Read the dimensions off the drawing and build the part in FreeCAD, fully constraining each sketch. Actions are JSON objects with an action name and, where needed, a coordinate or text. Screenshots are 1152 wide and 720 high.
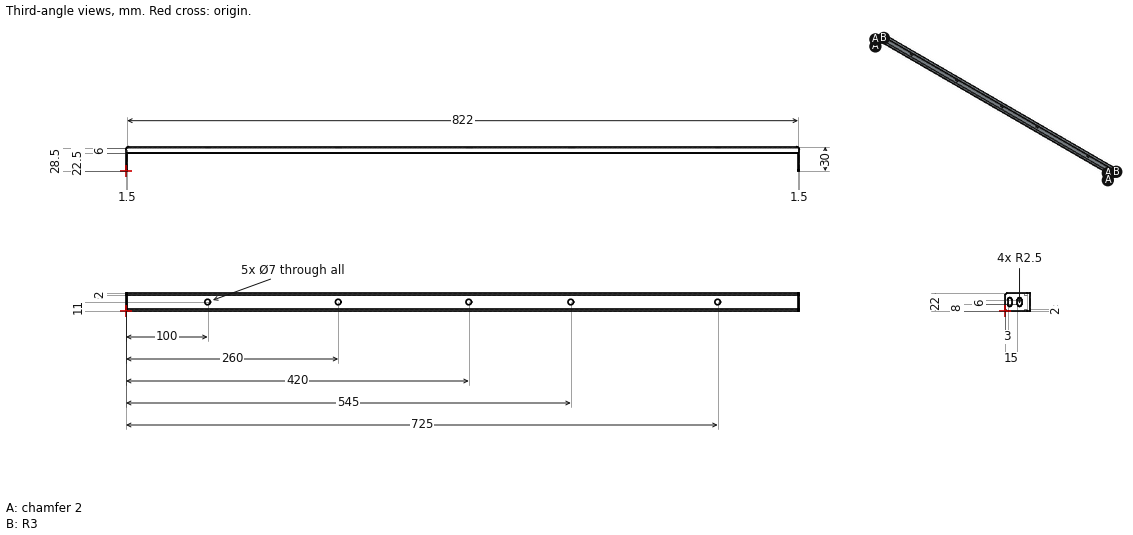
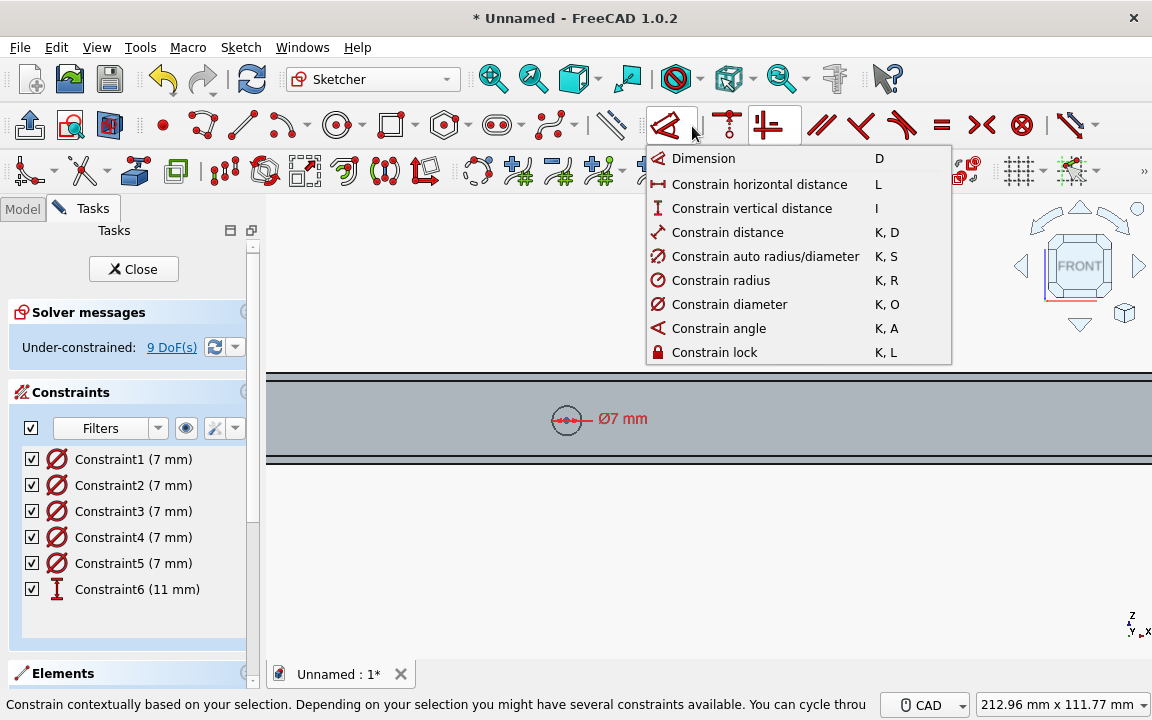
{"action": "left_click", "coordinate": [799, 208]}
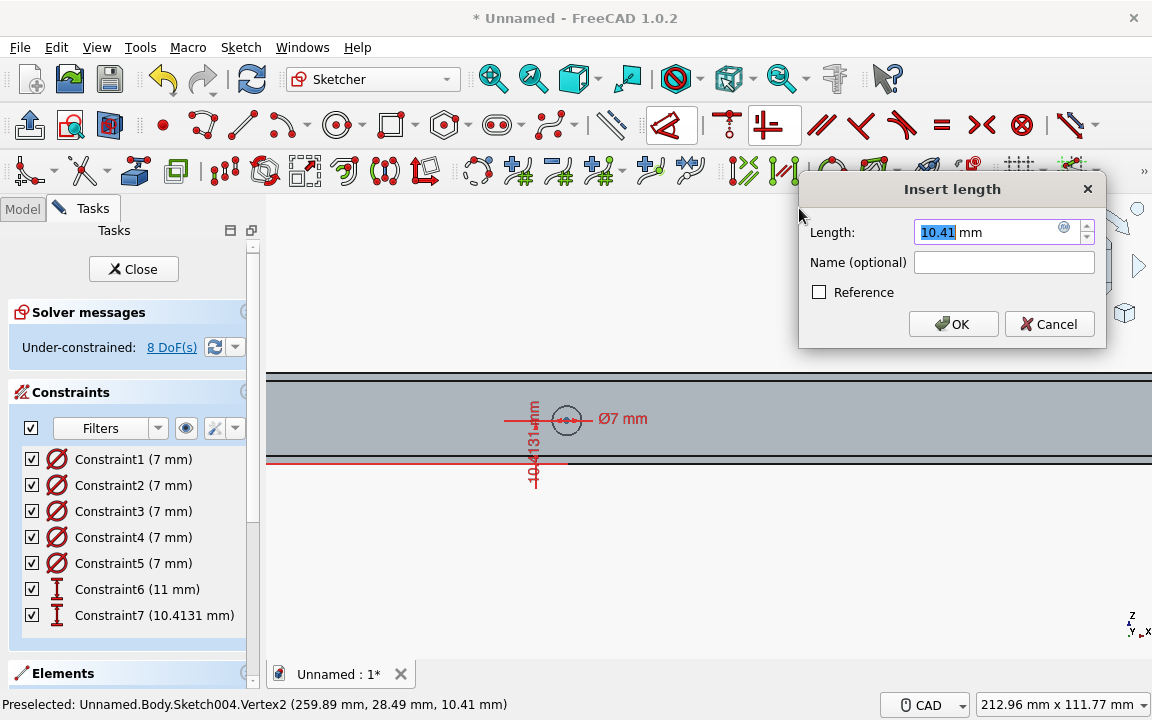
{"action": "type", "text": "11"}
{"action": "key", "text": "Return"}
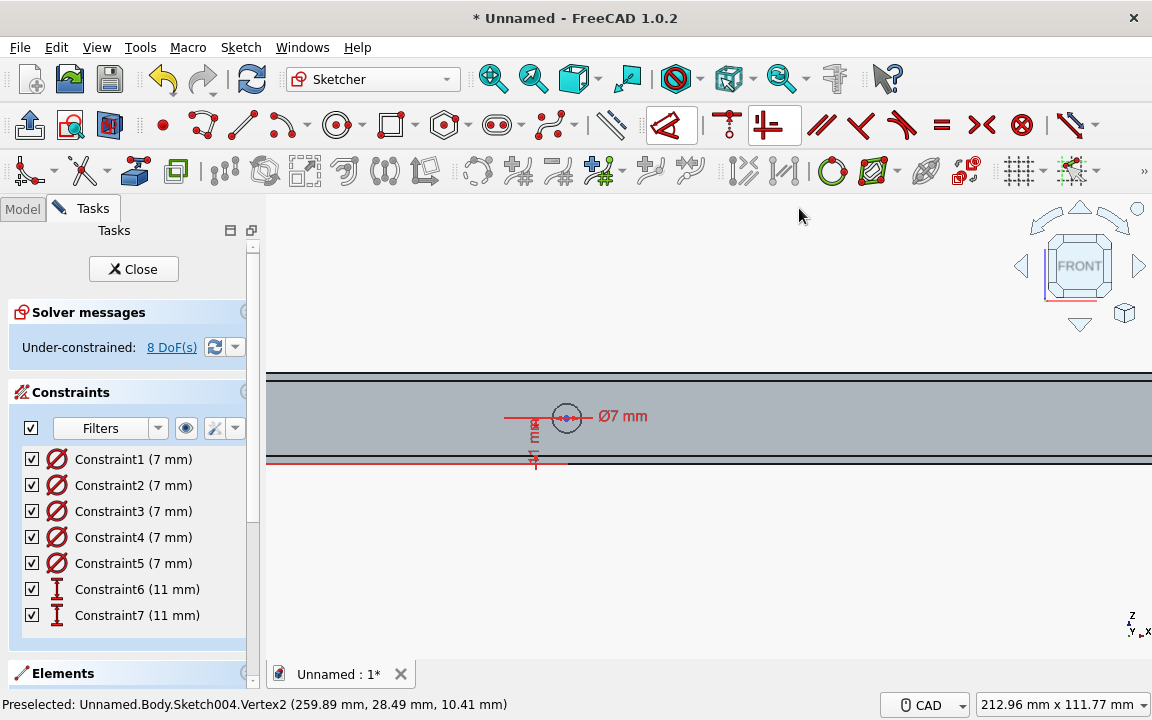
{"action": "scroll", "coordinate": [569, 425], "scroll_direction": "down", "scroll_amount": 9}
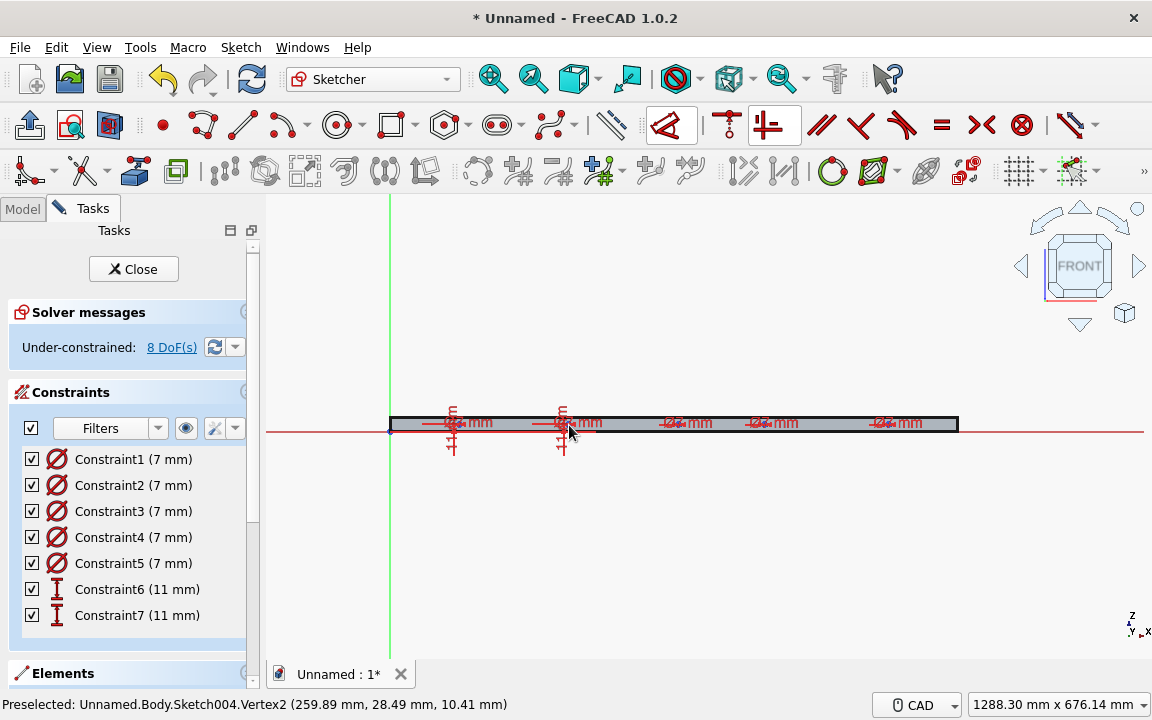
{"action": "scroll", "coordinate": [679, 425], "scroll_direction": "up", "scroll_amount": 9}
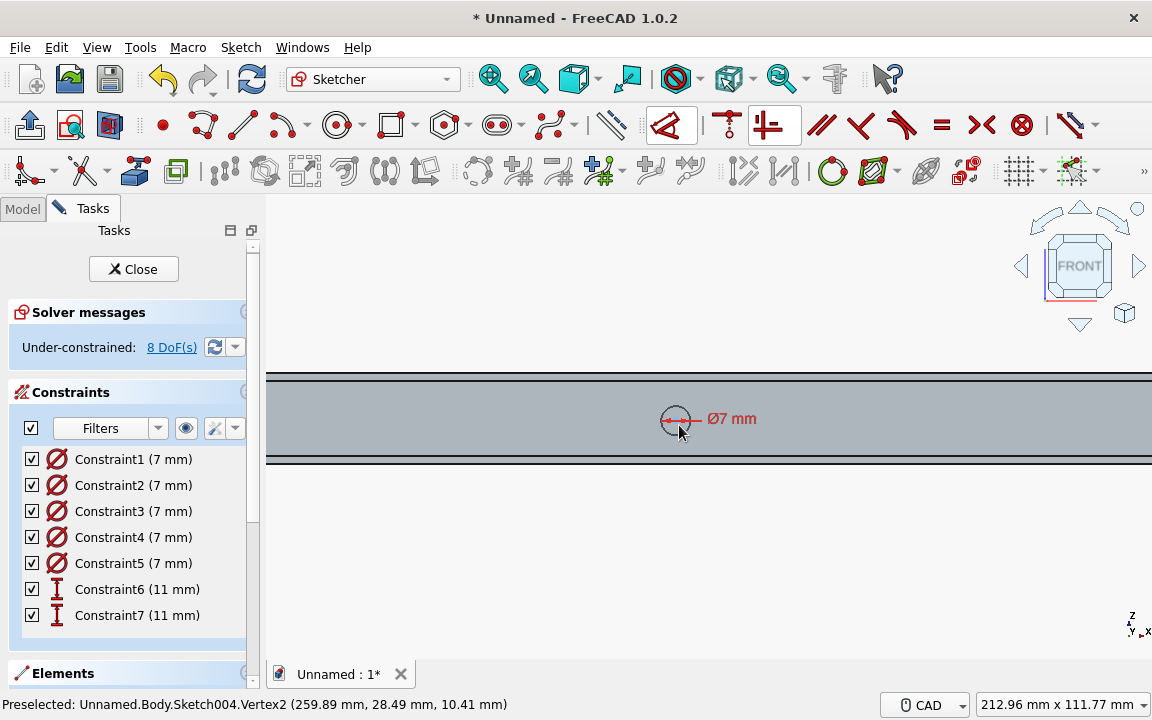
{"action": "left_click", "coordinate": [676, 421]}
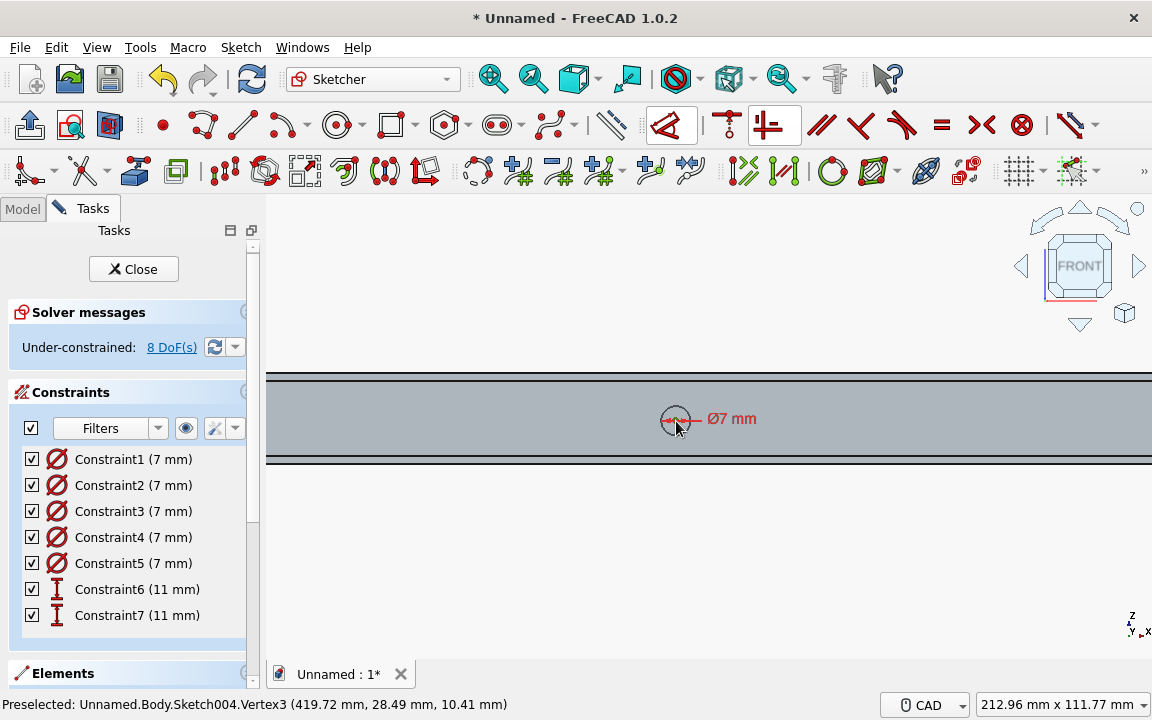
{"action": "left_click", "coordinate": [692, 126]}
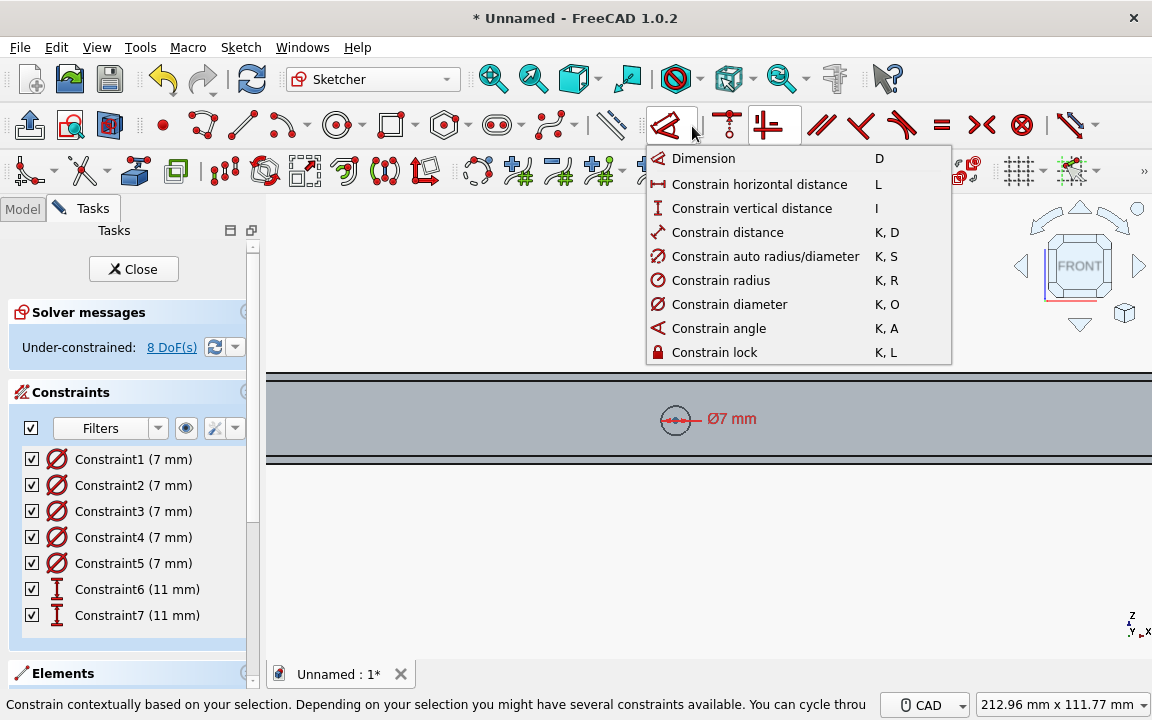
{"action": "left_click", "coordinate": [799, 208]}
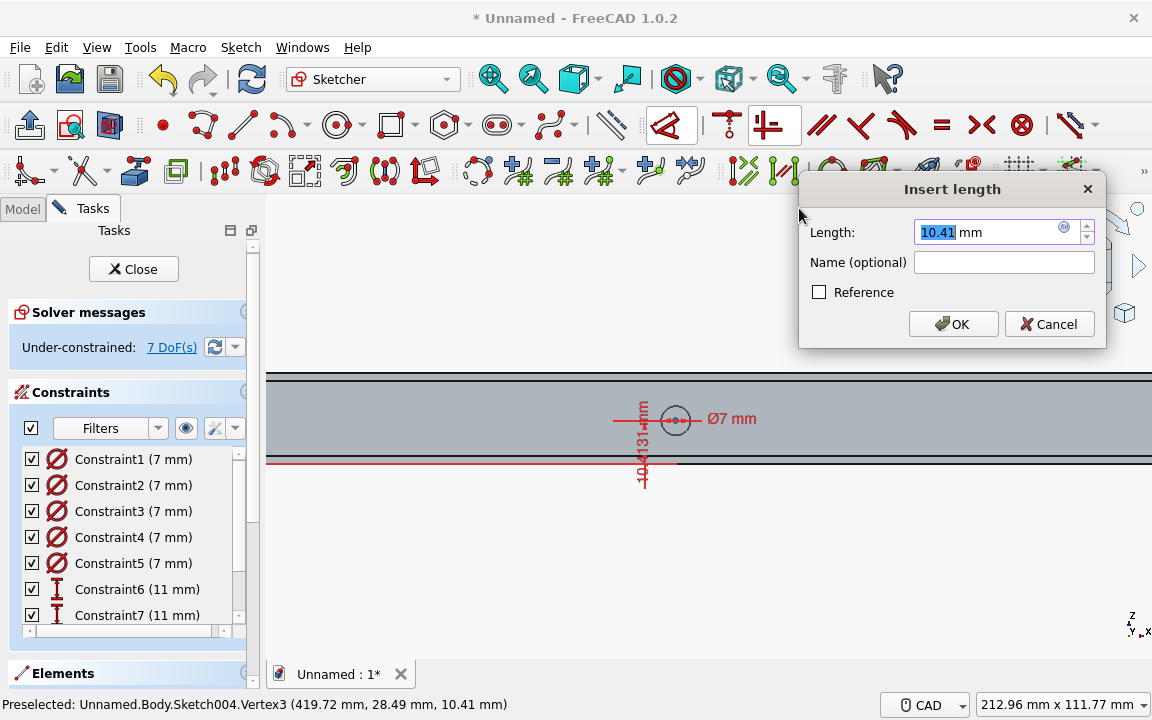
{"action": "type", "text": "11"}
{"action": "key", "text": "Return"}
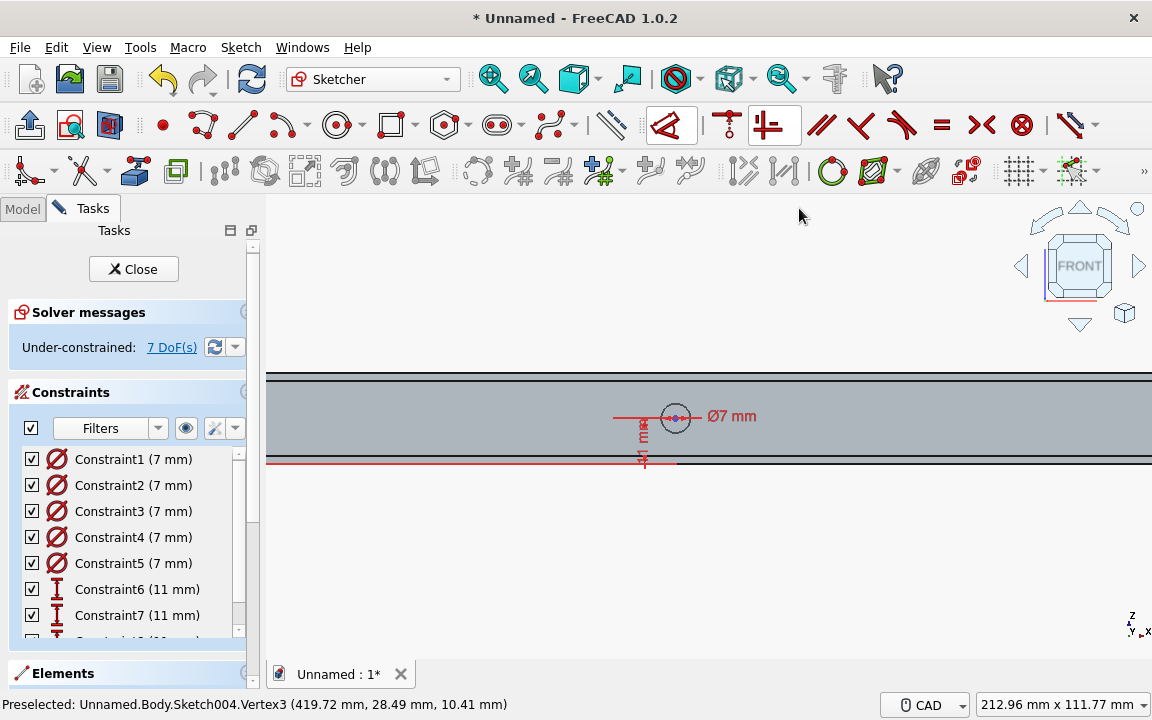
{"action": "scroll", "coordinate": [679, 425], "scroll_direction": "down", "scroll_amount": 9}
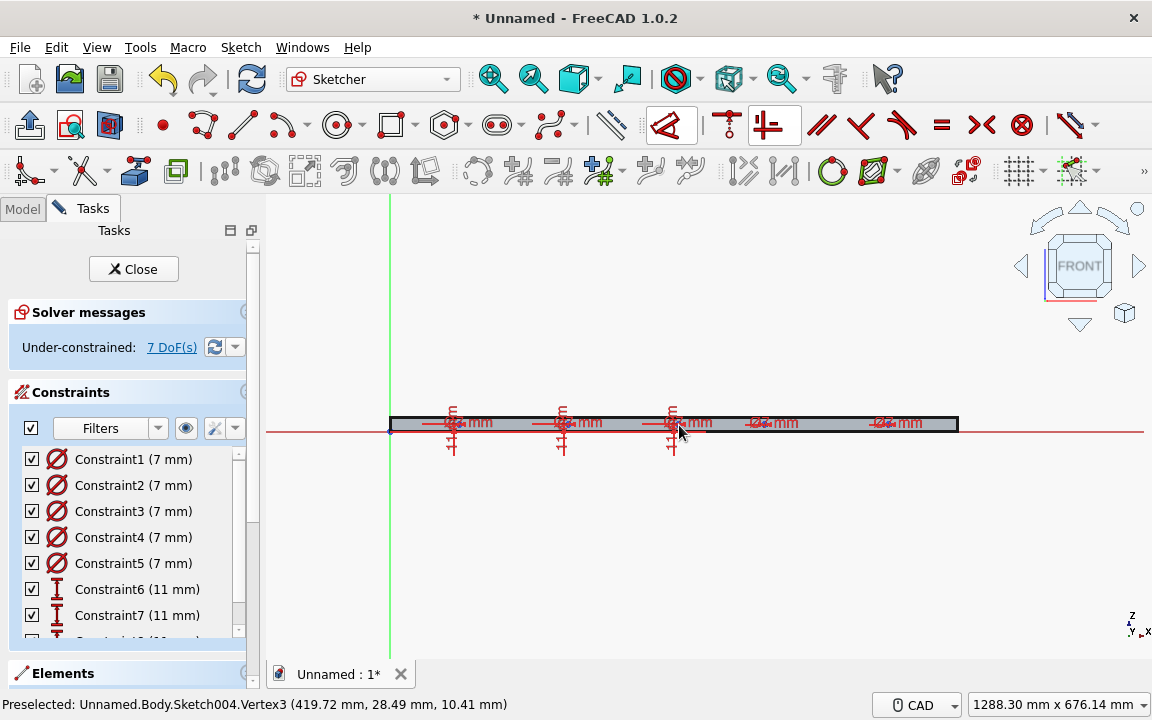
{"action": "scroll", "coordinate": [765, 425], "scroll_direction": "up", "scroll_amount": 9}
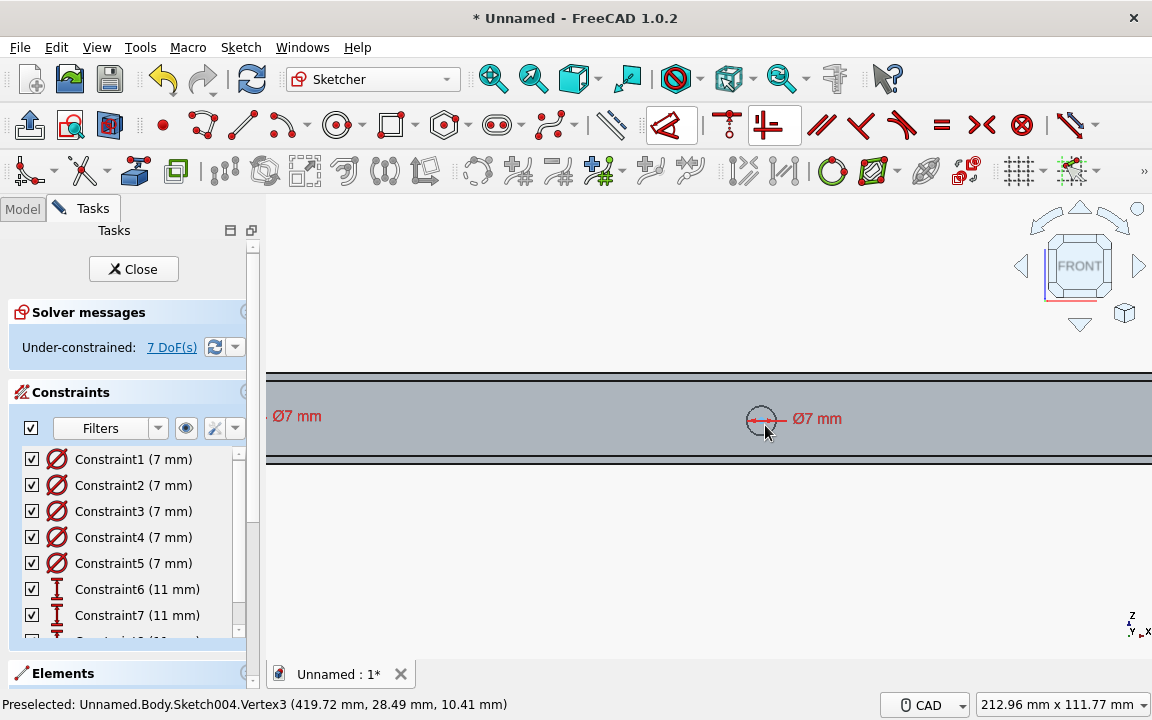
{"action": "left_click", "coordinate": [761, 421]}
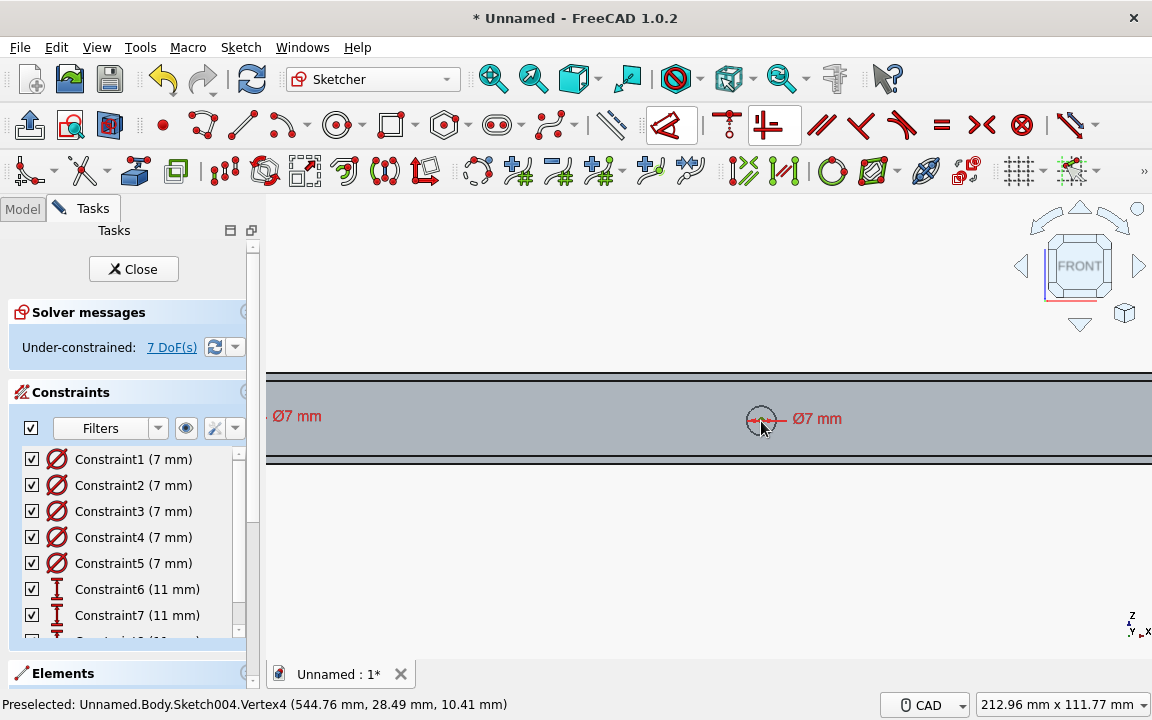
{"action": "left_click", "coordinate": [692, 126]}